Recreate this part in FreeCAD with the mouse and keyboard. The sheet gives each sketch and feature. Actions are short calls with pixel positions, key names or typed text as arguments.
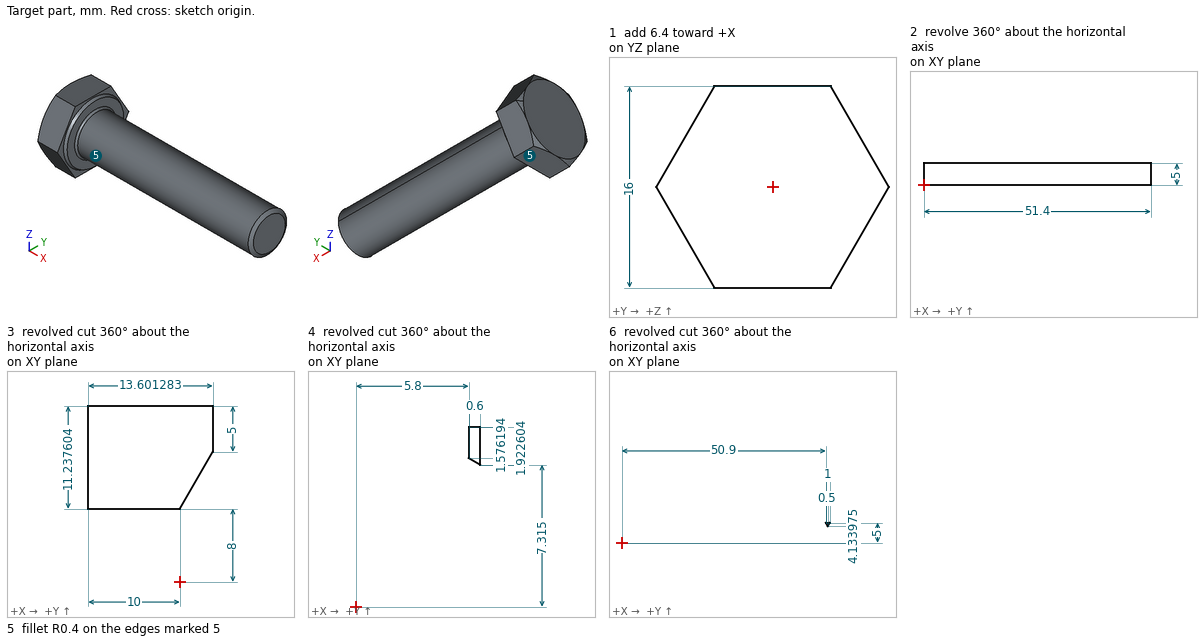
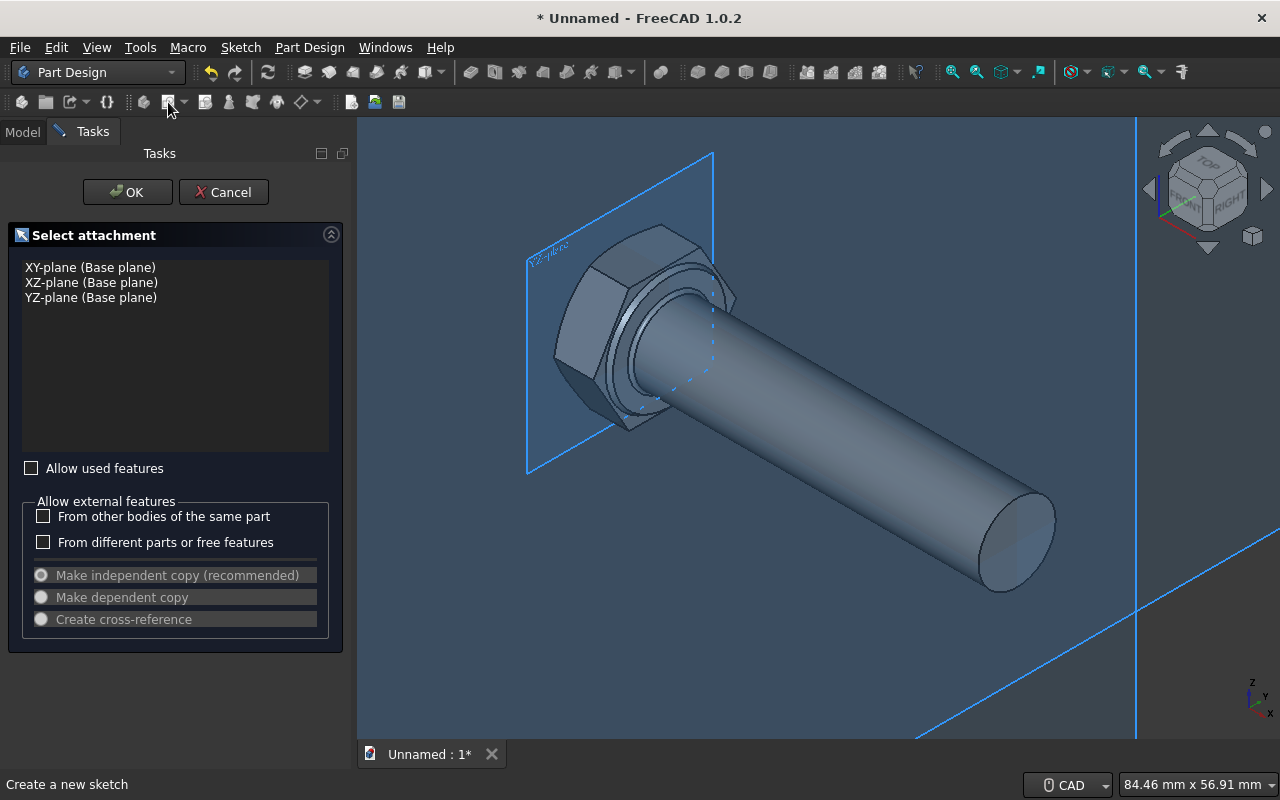
click(82, 268)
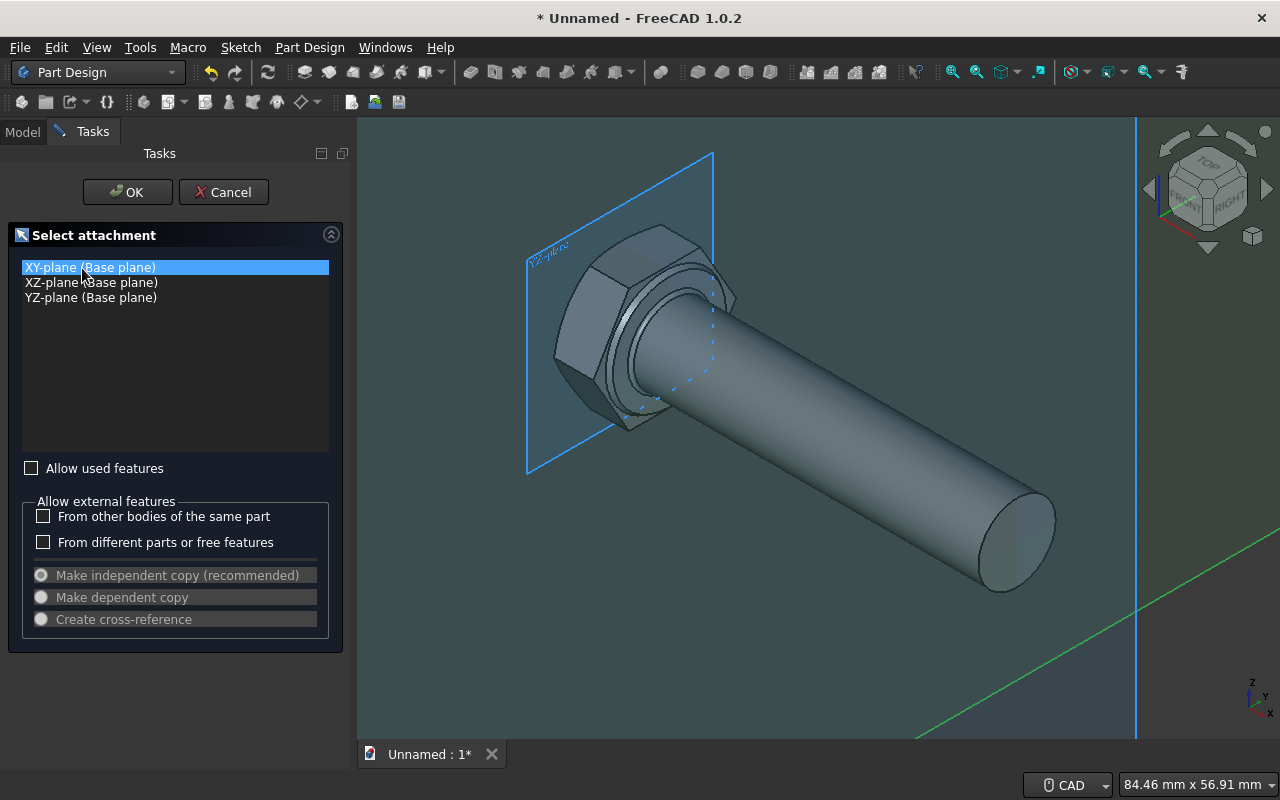
click(128, 192)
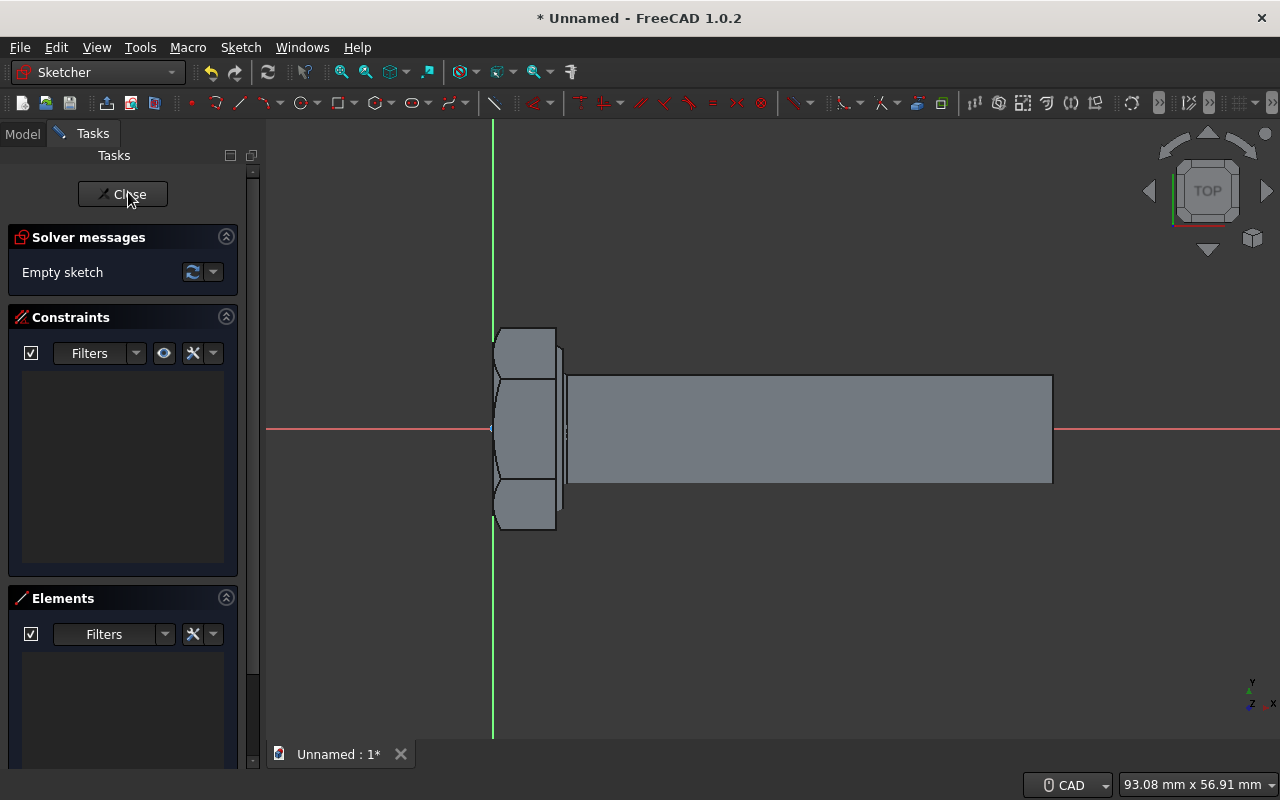
click(156, 104)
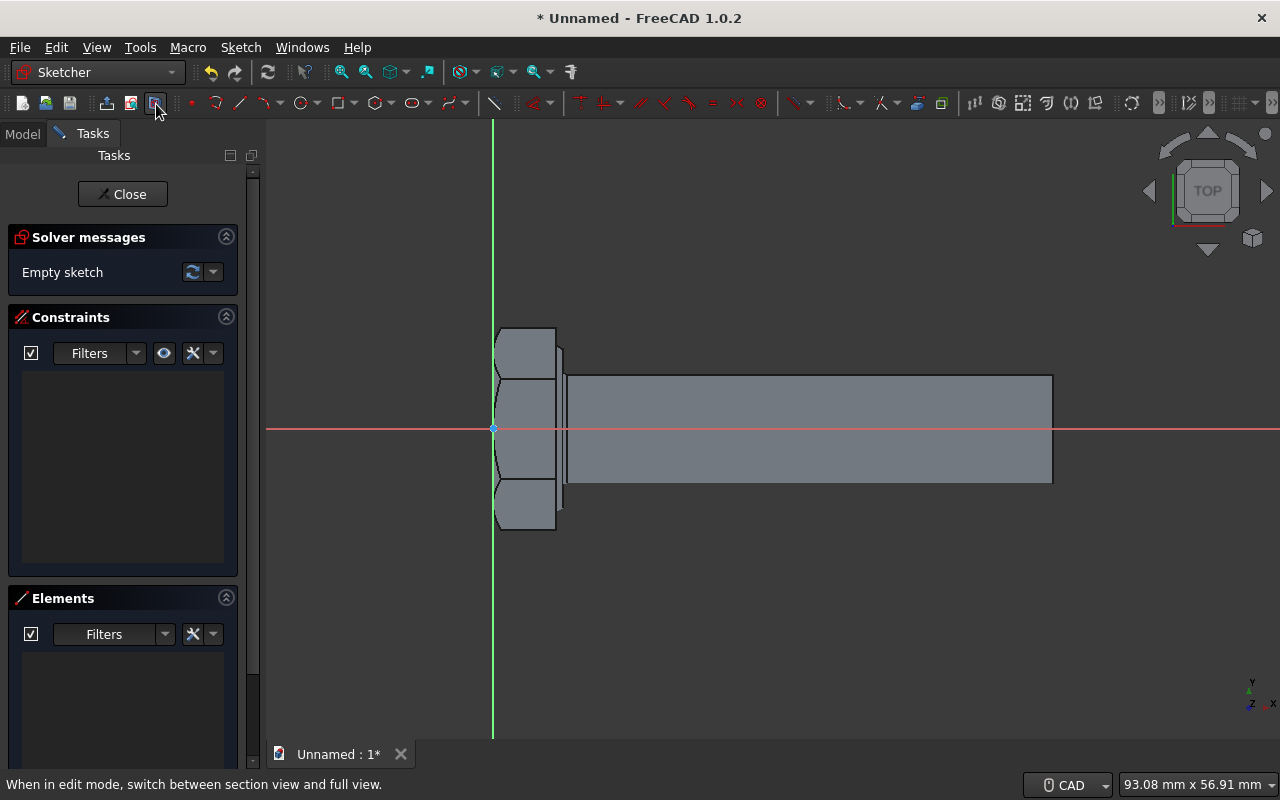
scroll(1071, 377, up, 15)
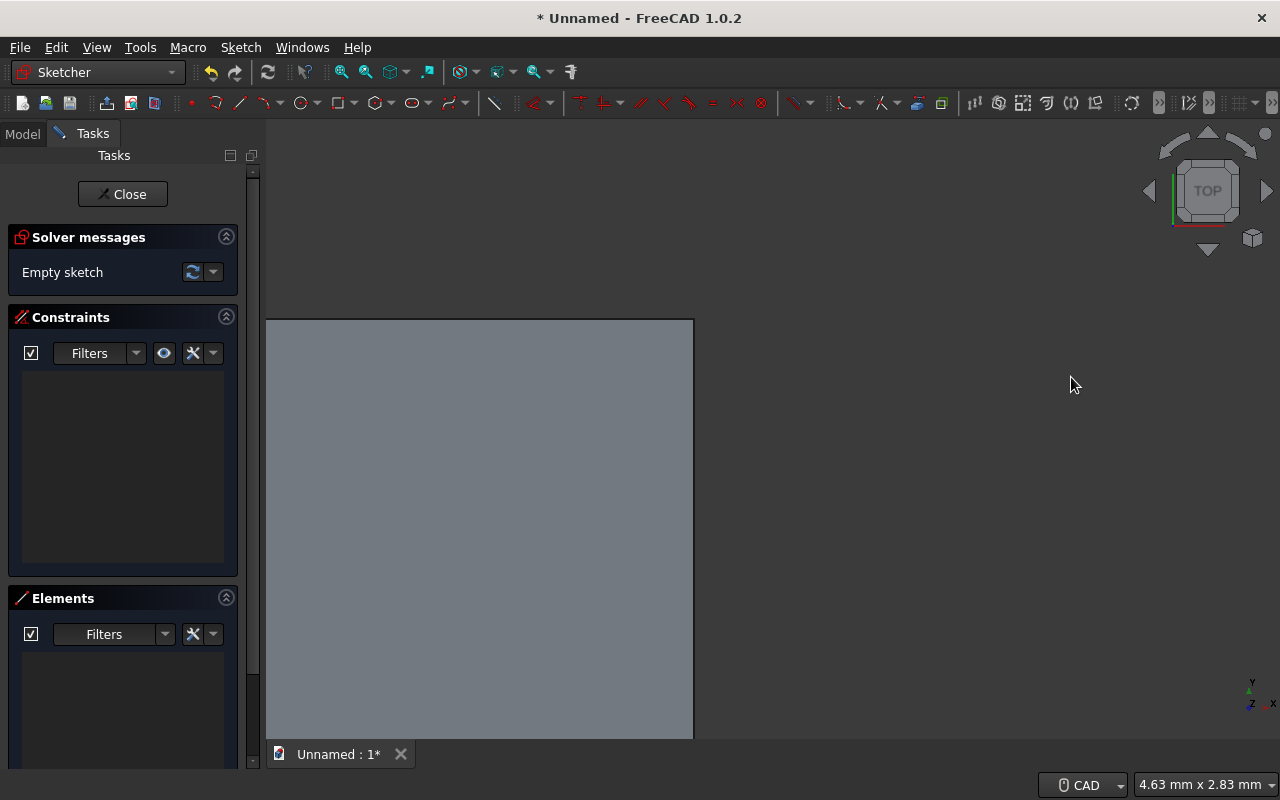
scroll(685, 402, up, 4)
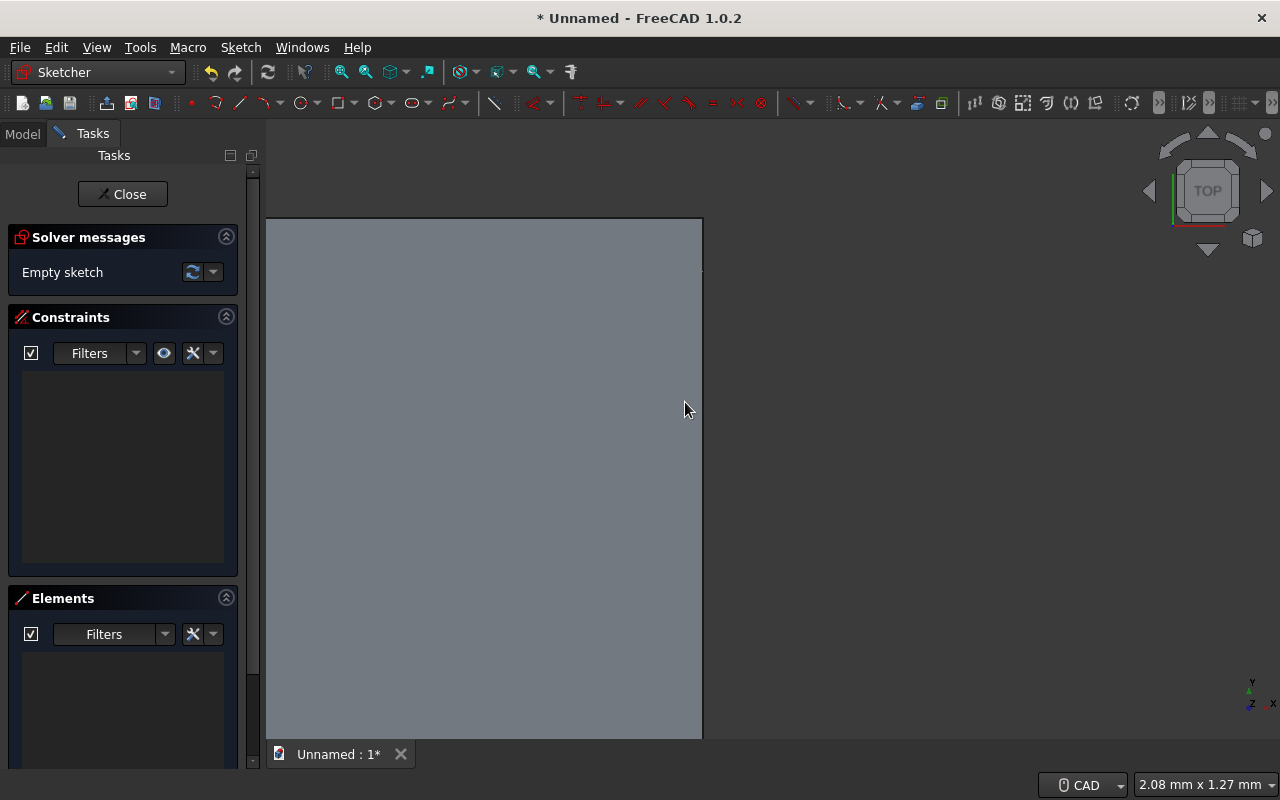
key(g)
key(m)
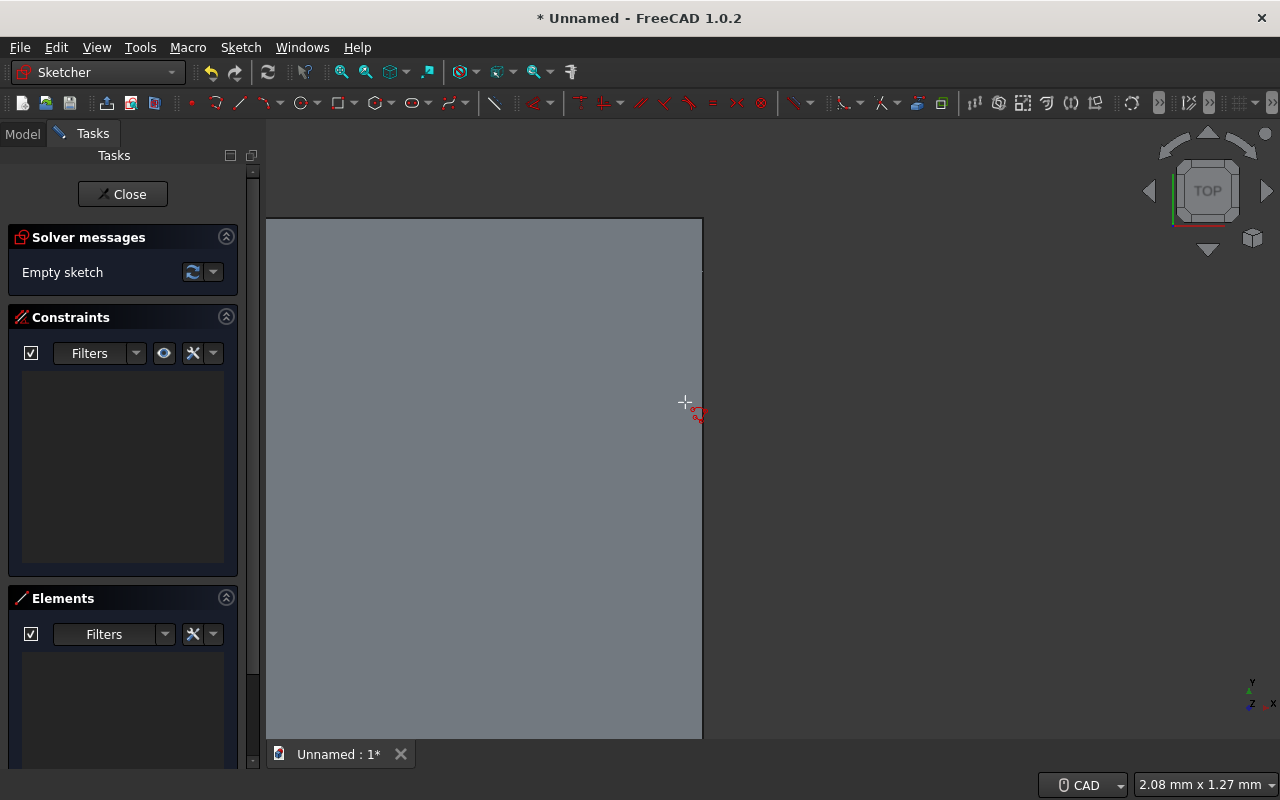
click(460, 218)
click(703, 640)
click(947, 218)
click(460, 219)
key(Escape)
key(Escape)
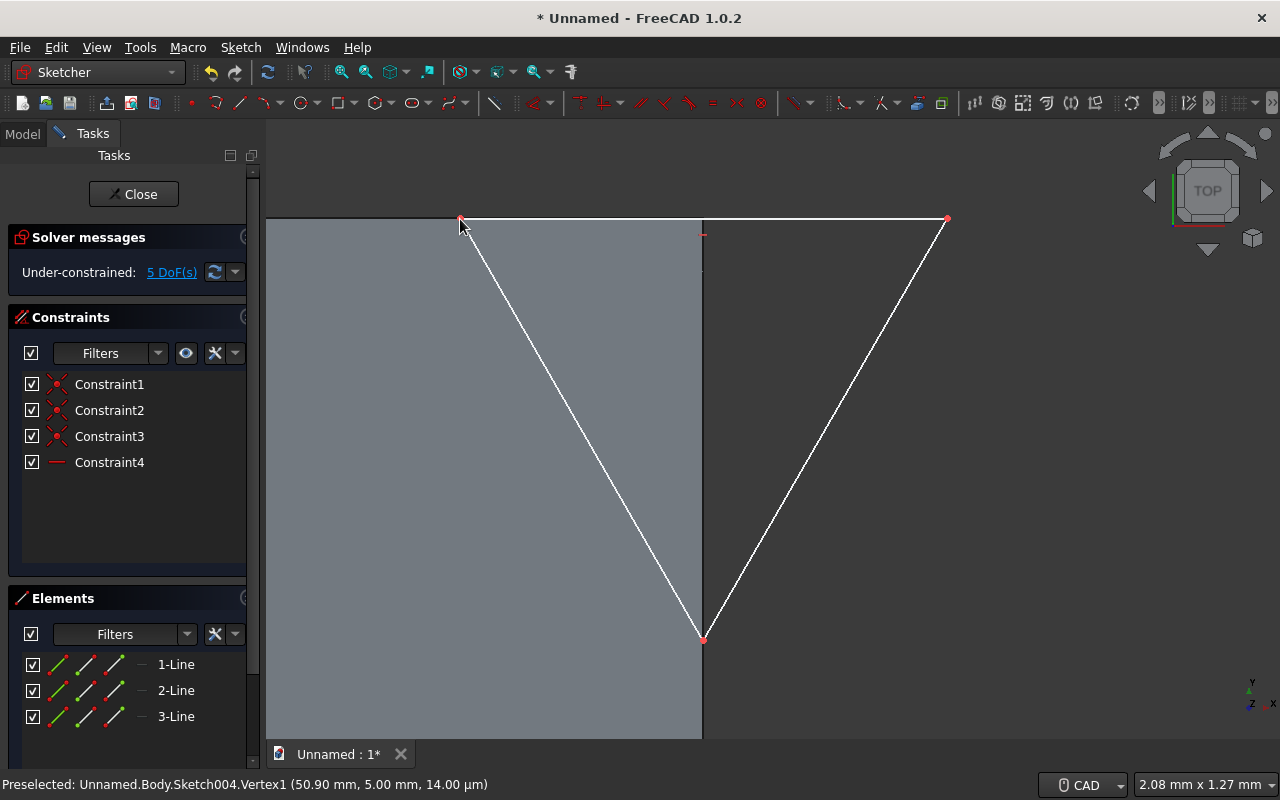
click(534, 104)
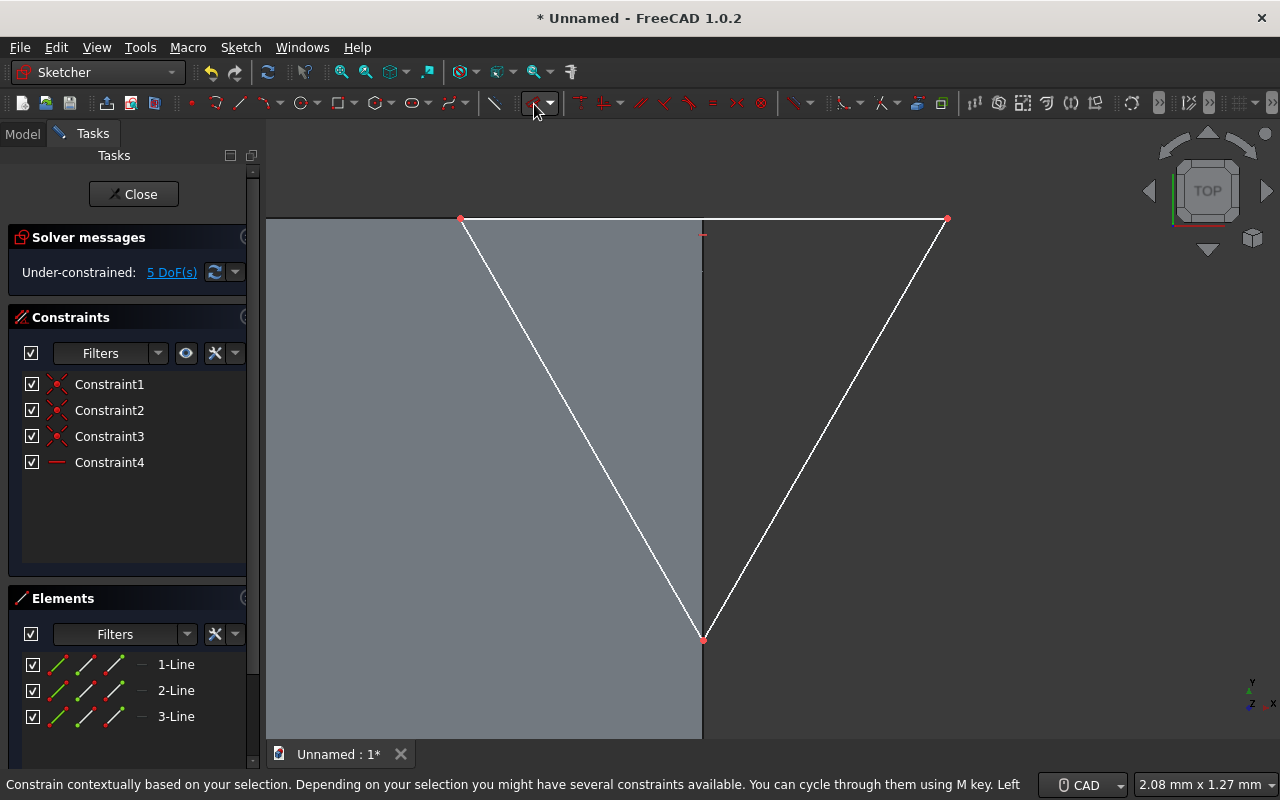
click(801, 219)
click(704, 185)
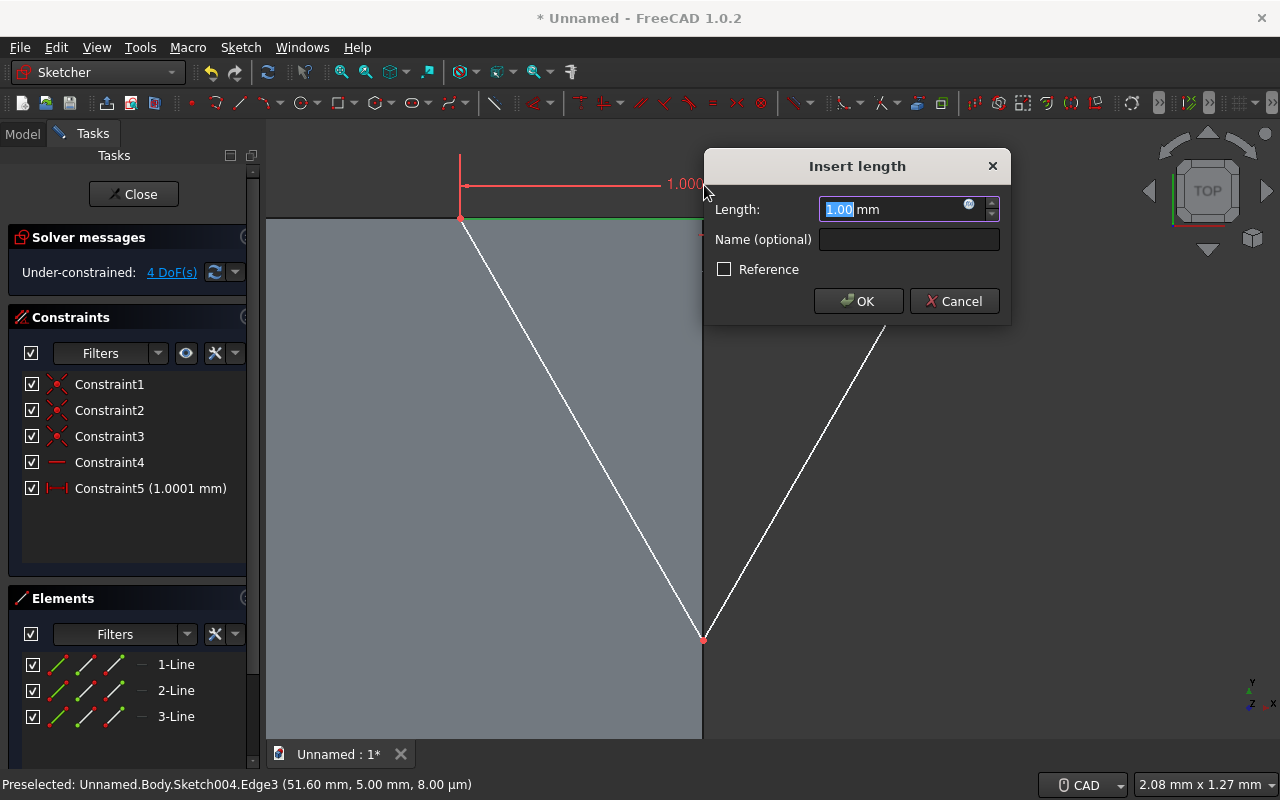
text(1)
key(Return)